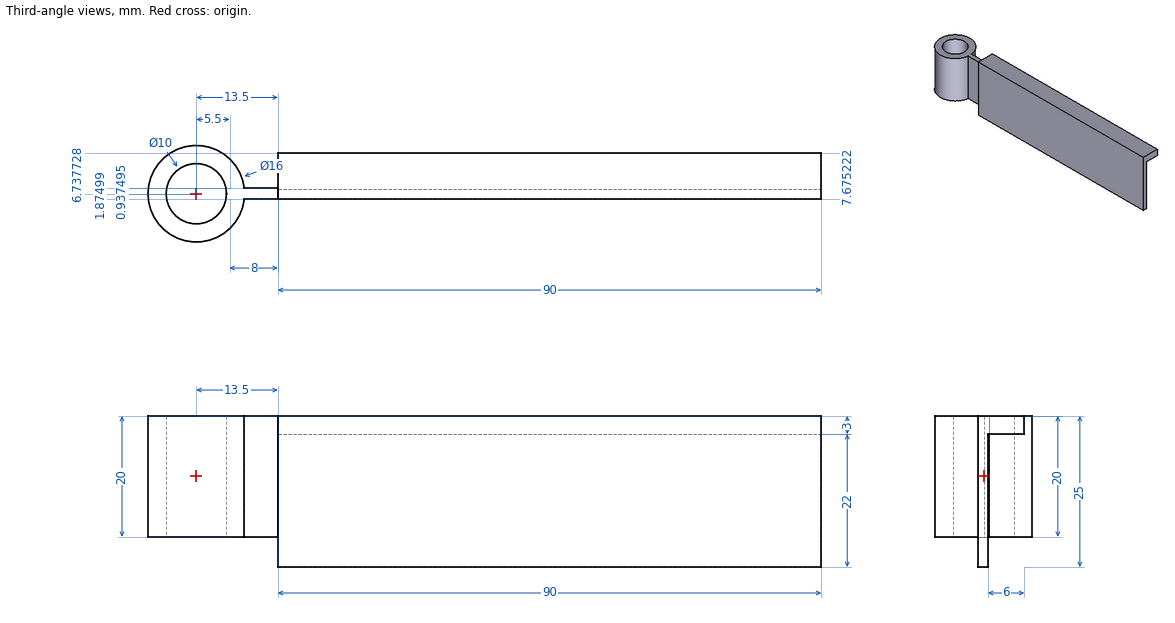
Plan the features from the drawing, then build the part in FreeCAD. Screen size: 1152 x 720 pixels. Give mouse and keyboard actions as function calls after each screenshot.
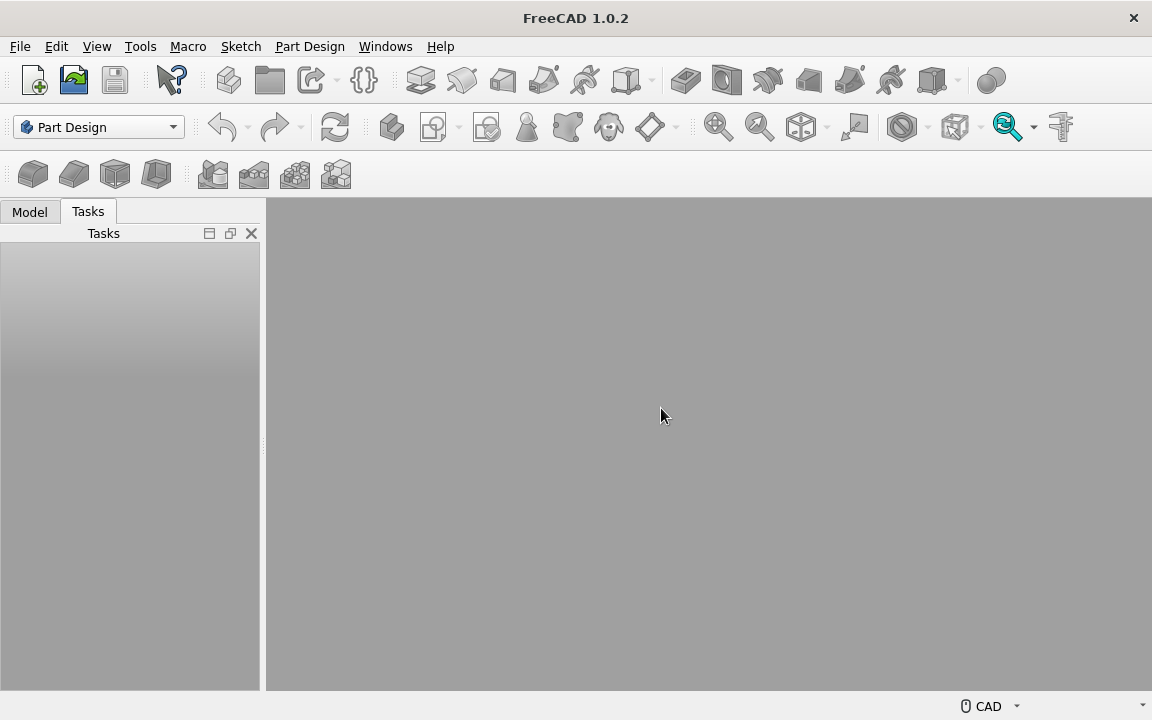
click(33, 80)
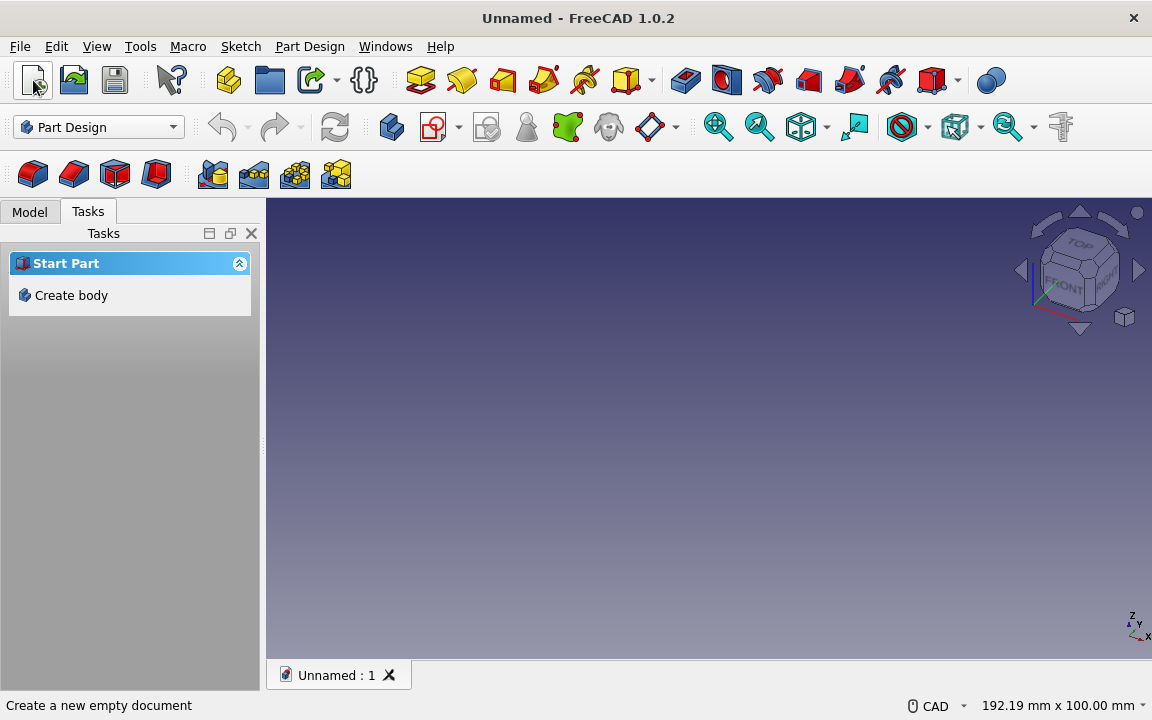
click(432, 128)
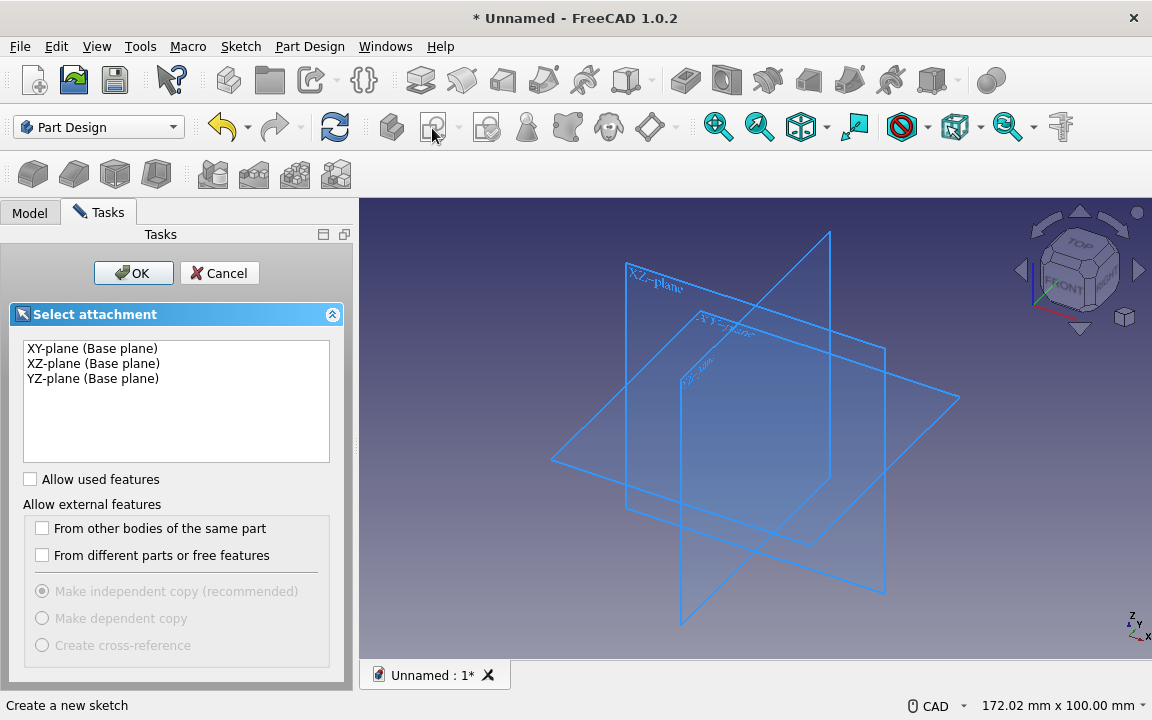
click(84, 348)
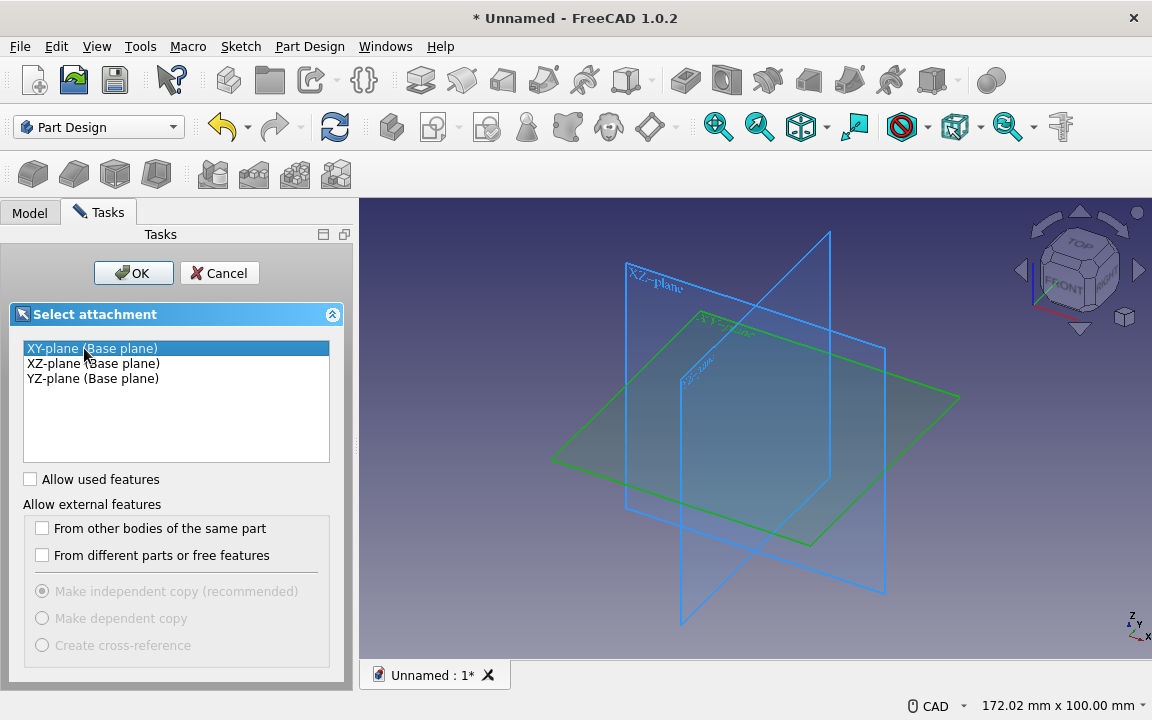
click(134, 273)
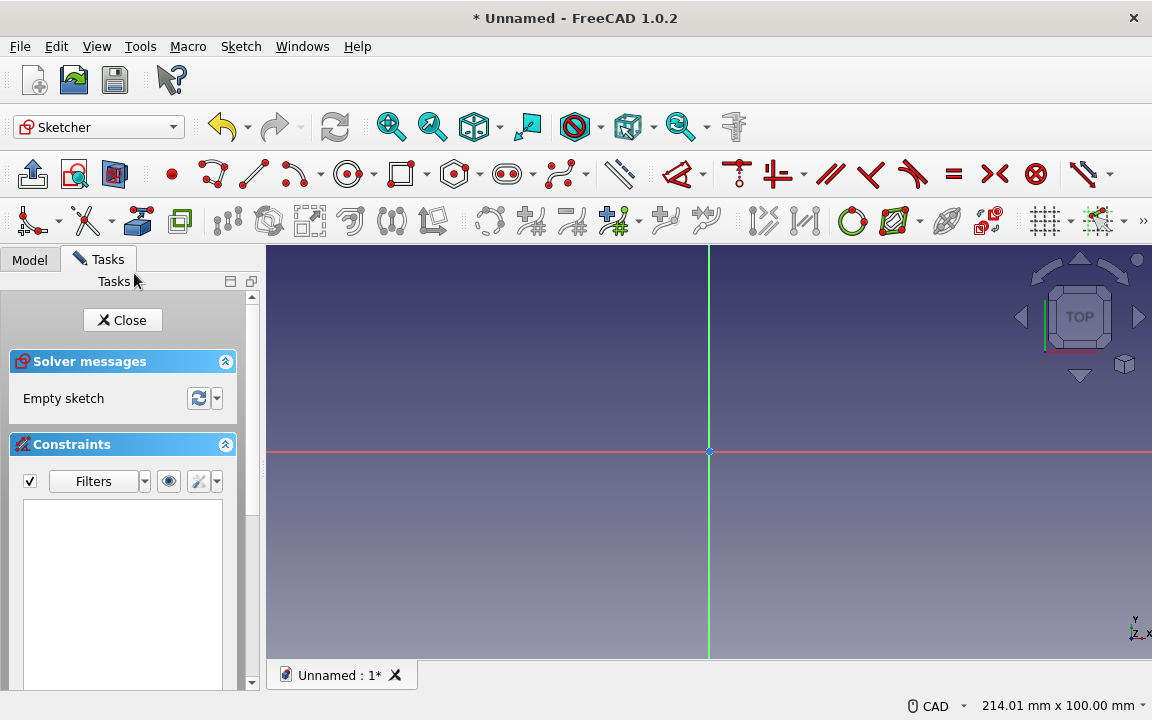
scroll(731, 452, up, 7)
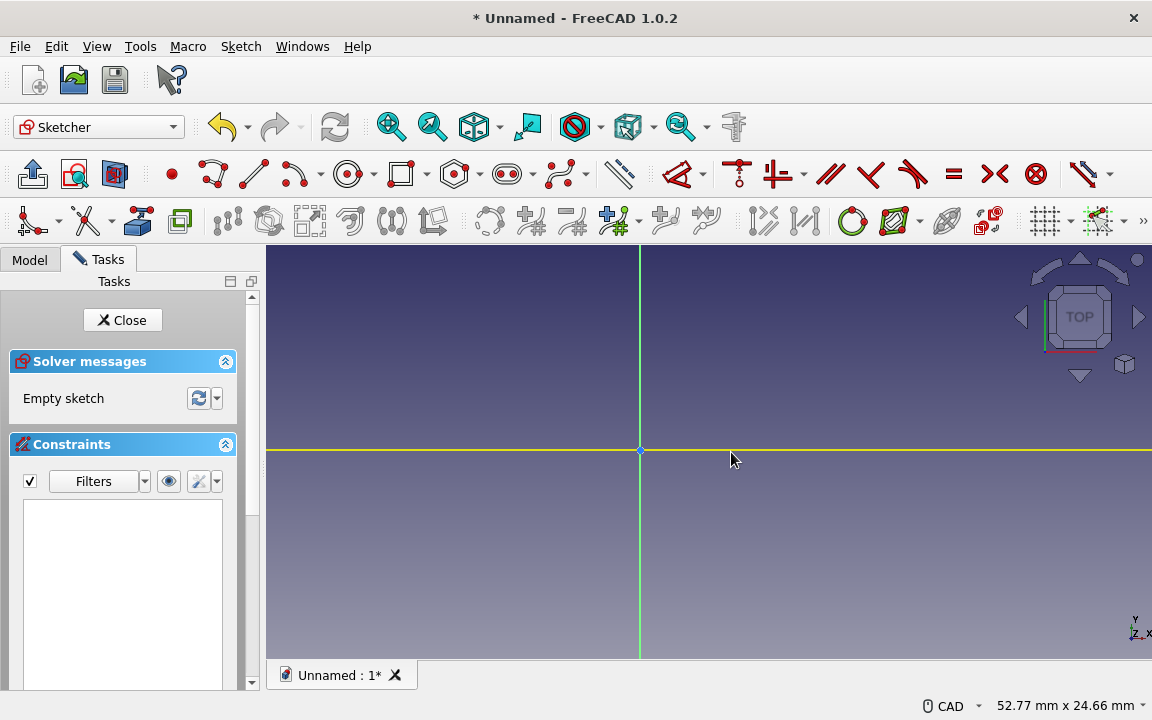
click(348, 174)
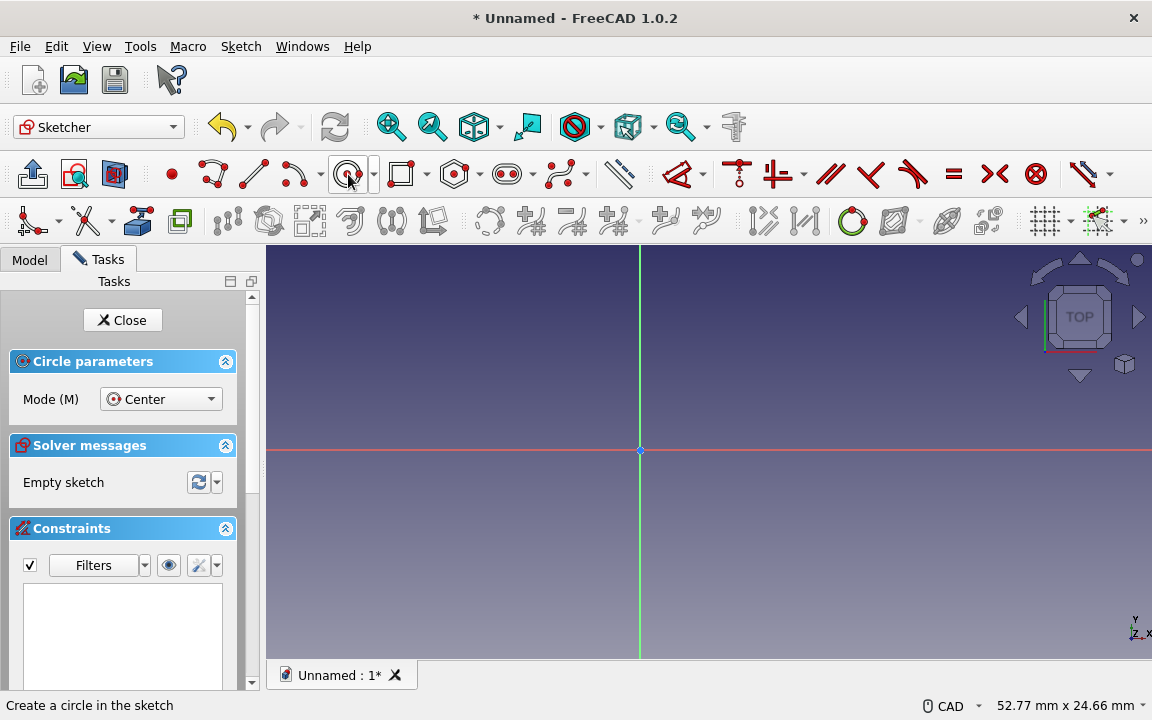
click(640, 450)
move(735, 355)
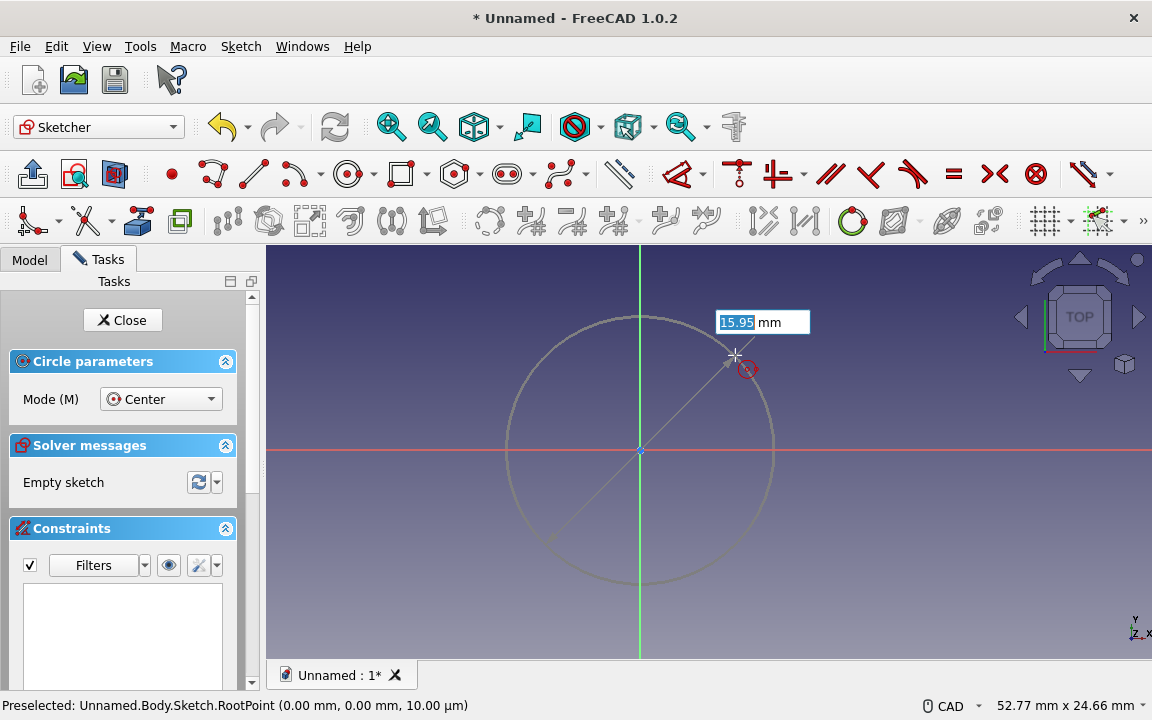
text(16)
key(Return)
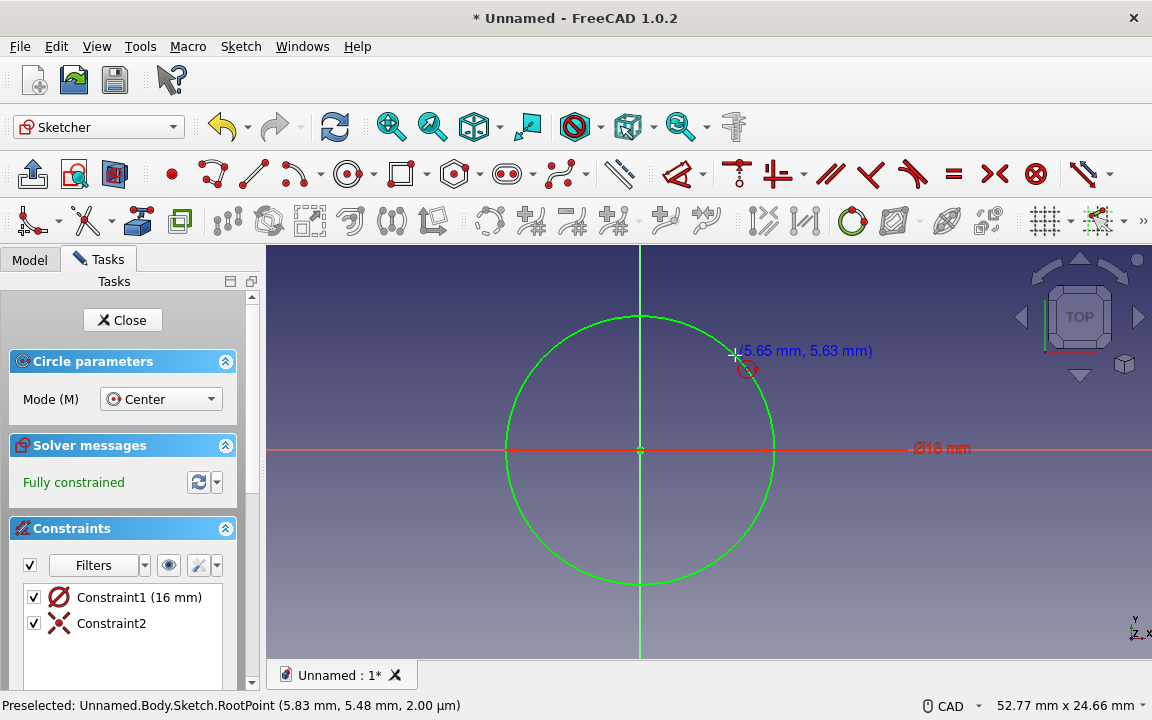
click(640, 450)
move(700, 391)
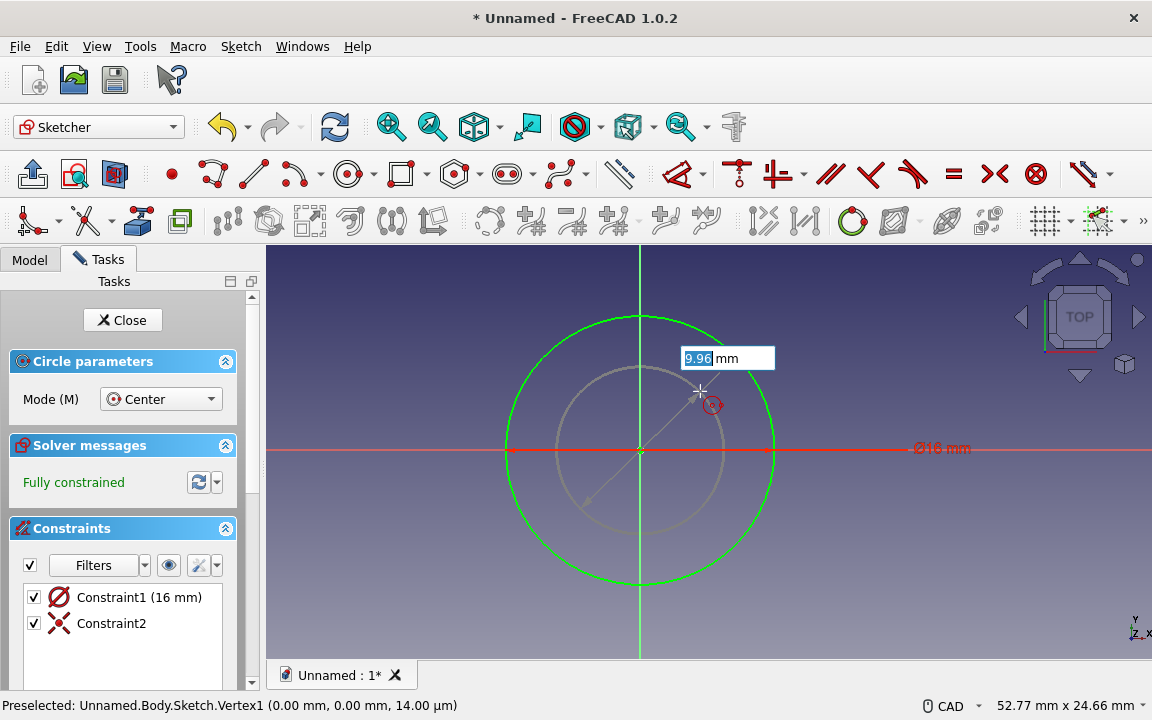
text(10)
key(Return)
key(Escape)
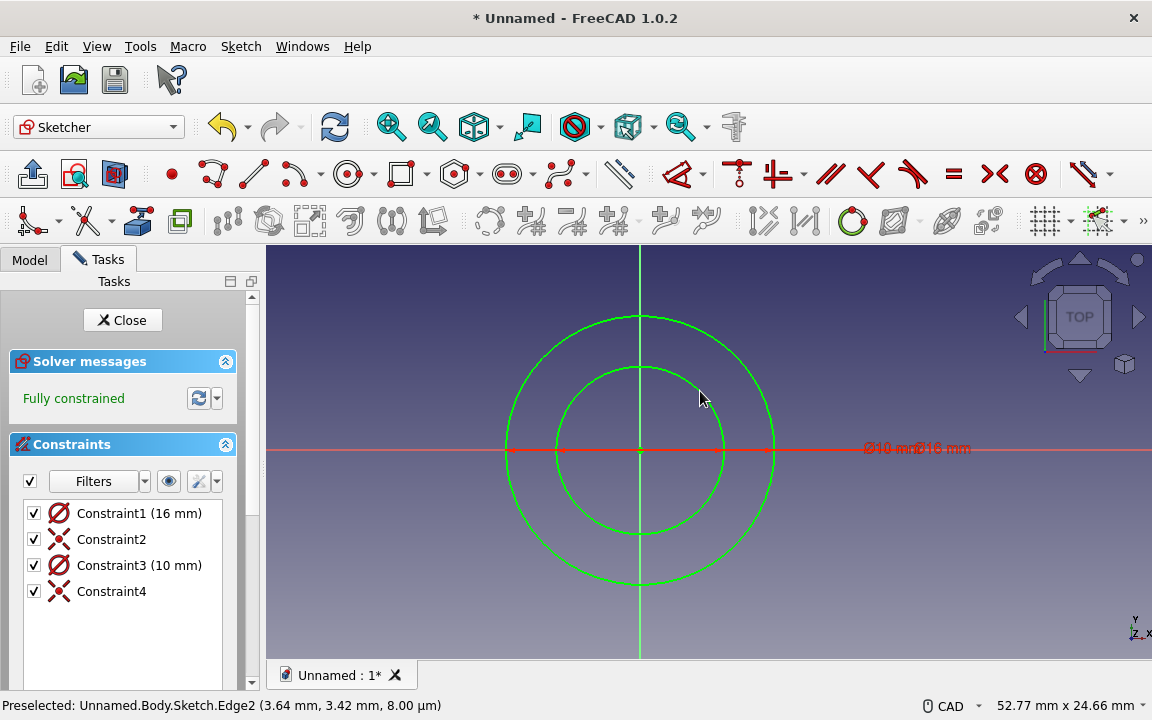
click(123, 320)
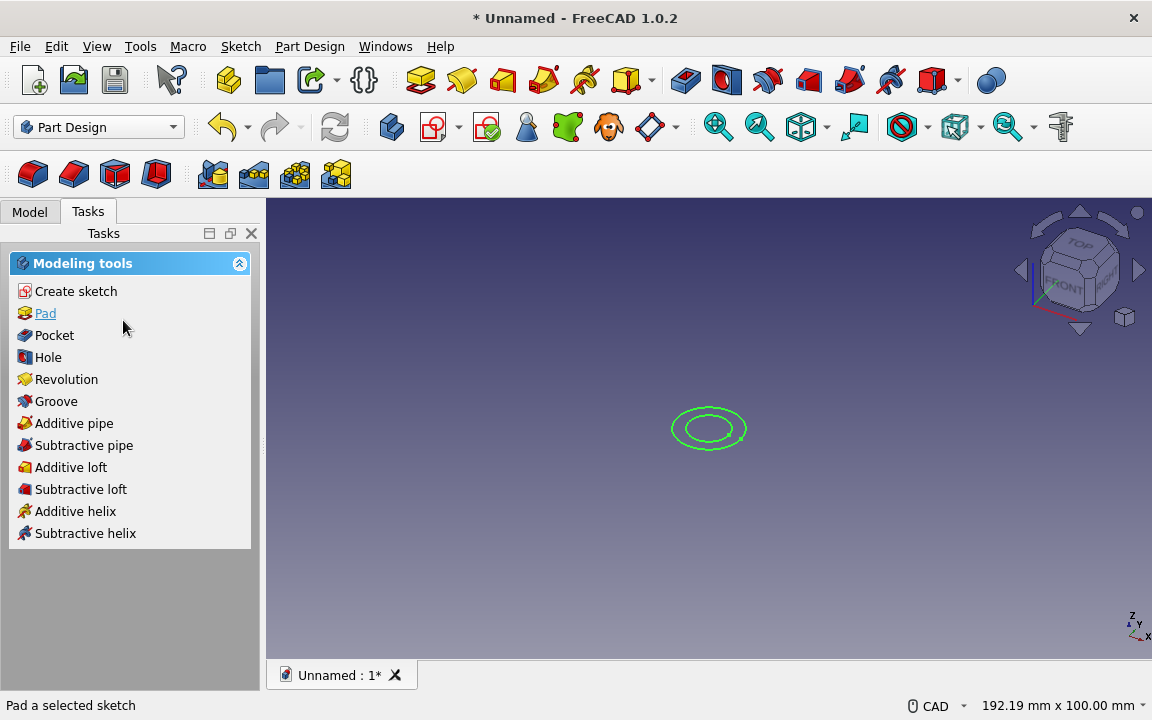
click(421, 80)